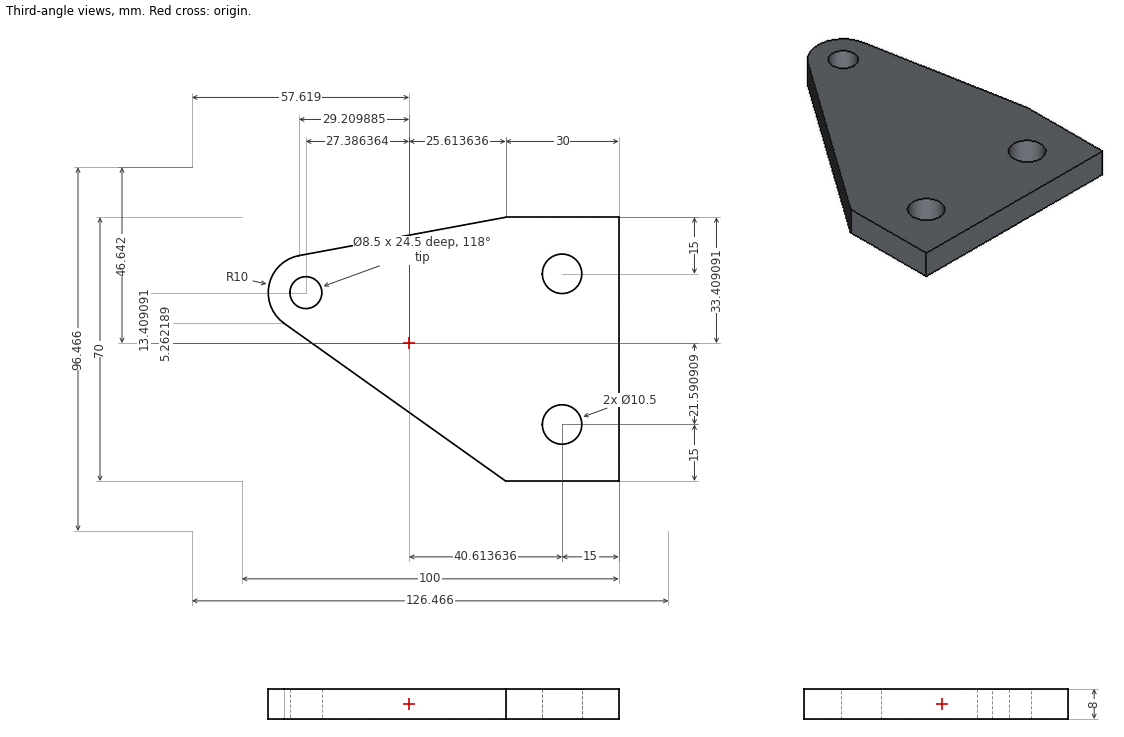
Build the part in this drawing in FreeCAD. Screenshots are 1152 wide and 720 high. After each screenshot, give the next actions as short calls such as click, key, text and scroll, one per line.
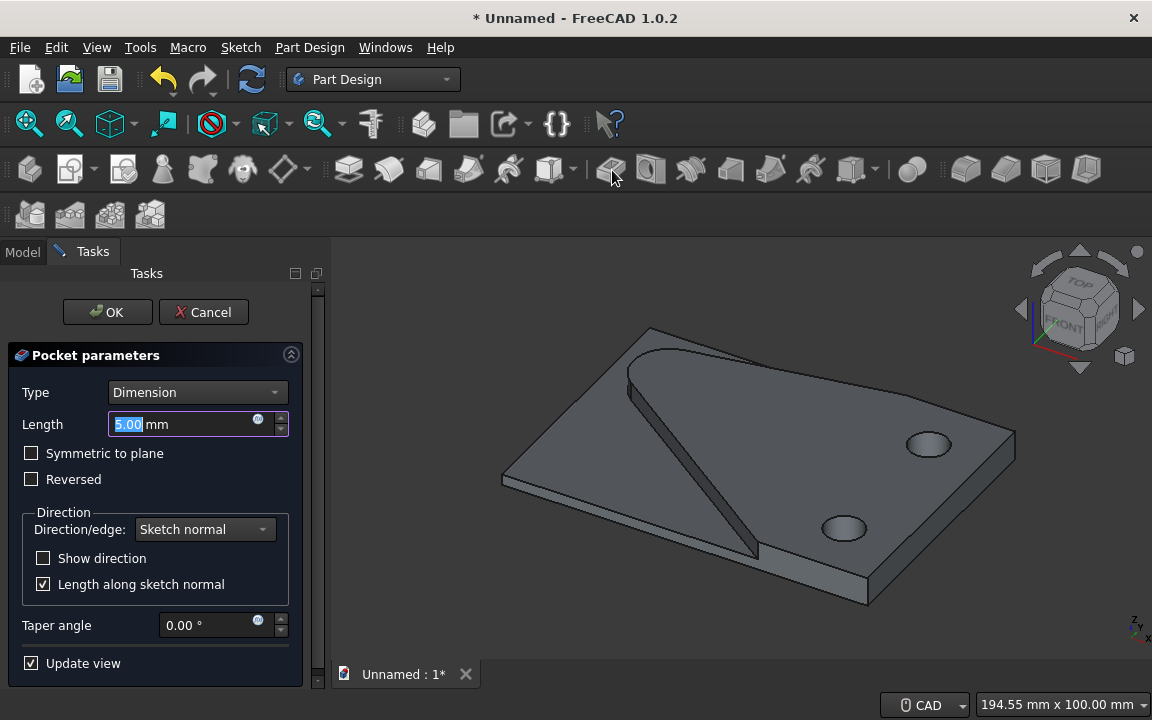
text(10)
key(Tab)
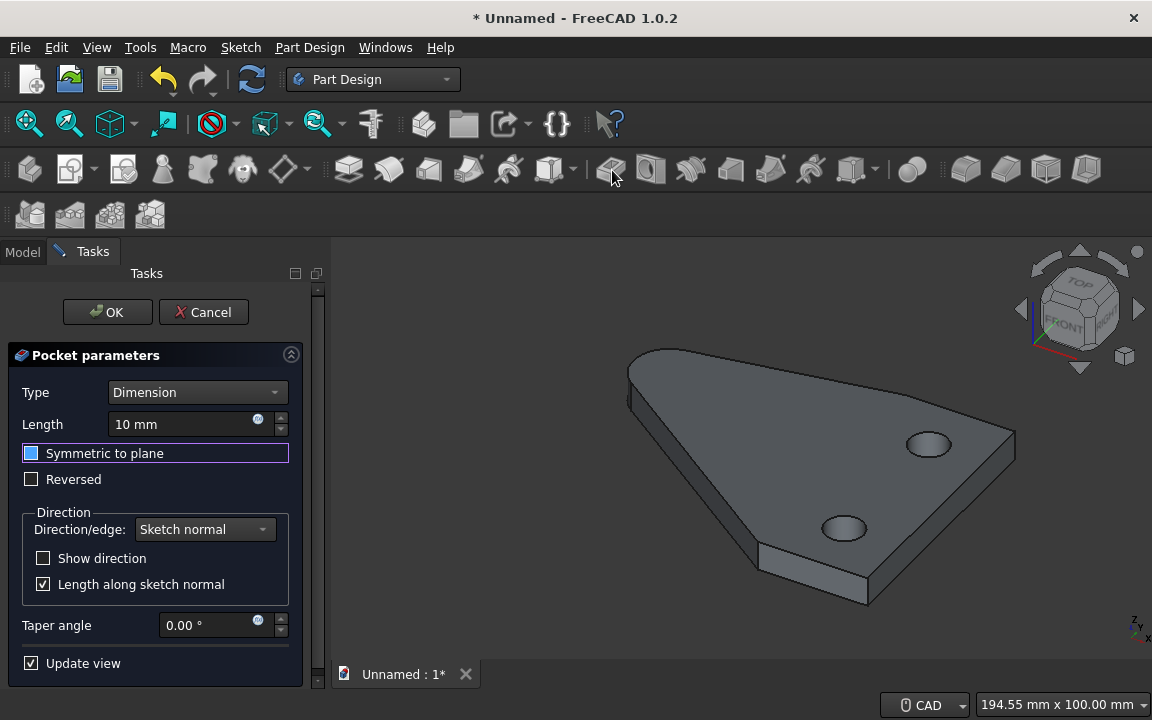
click(108, 312)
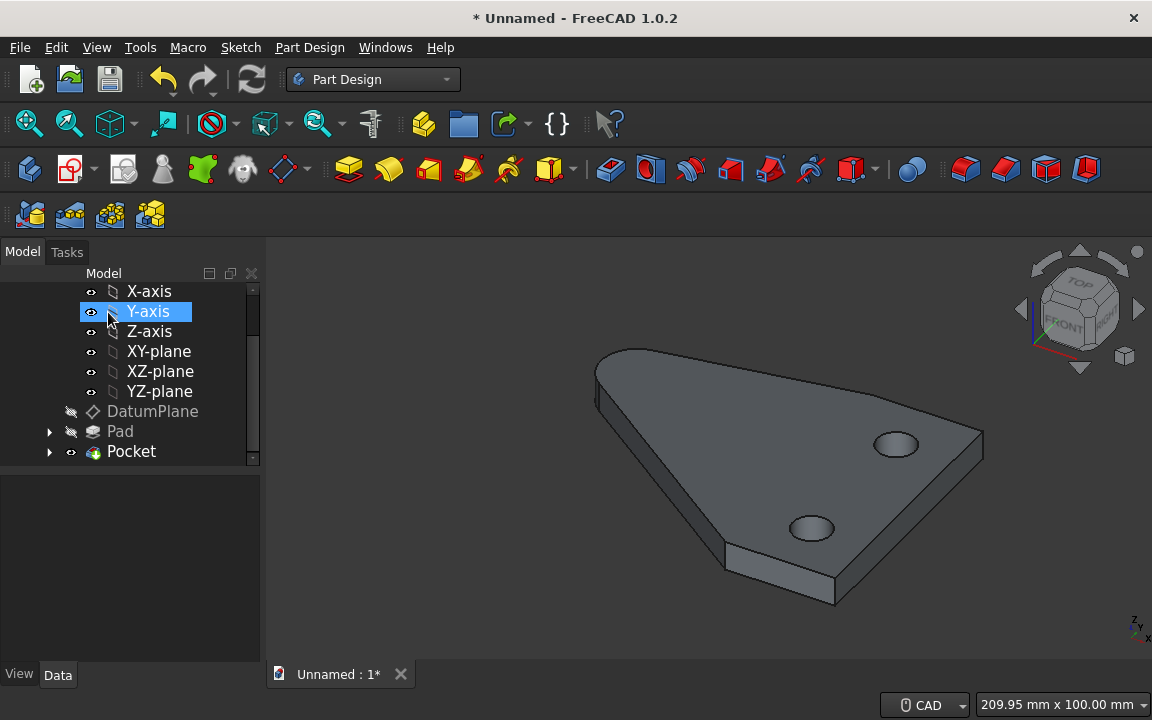
click(788, 464)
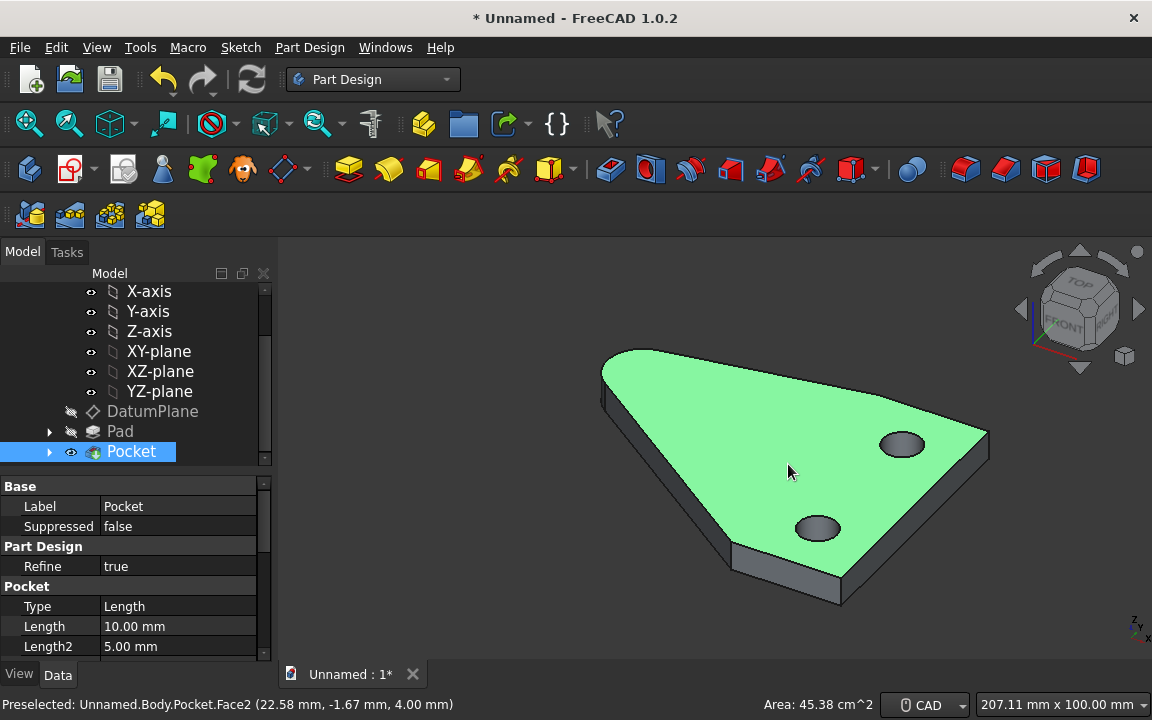
click(70, 170)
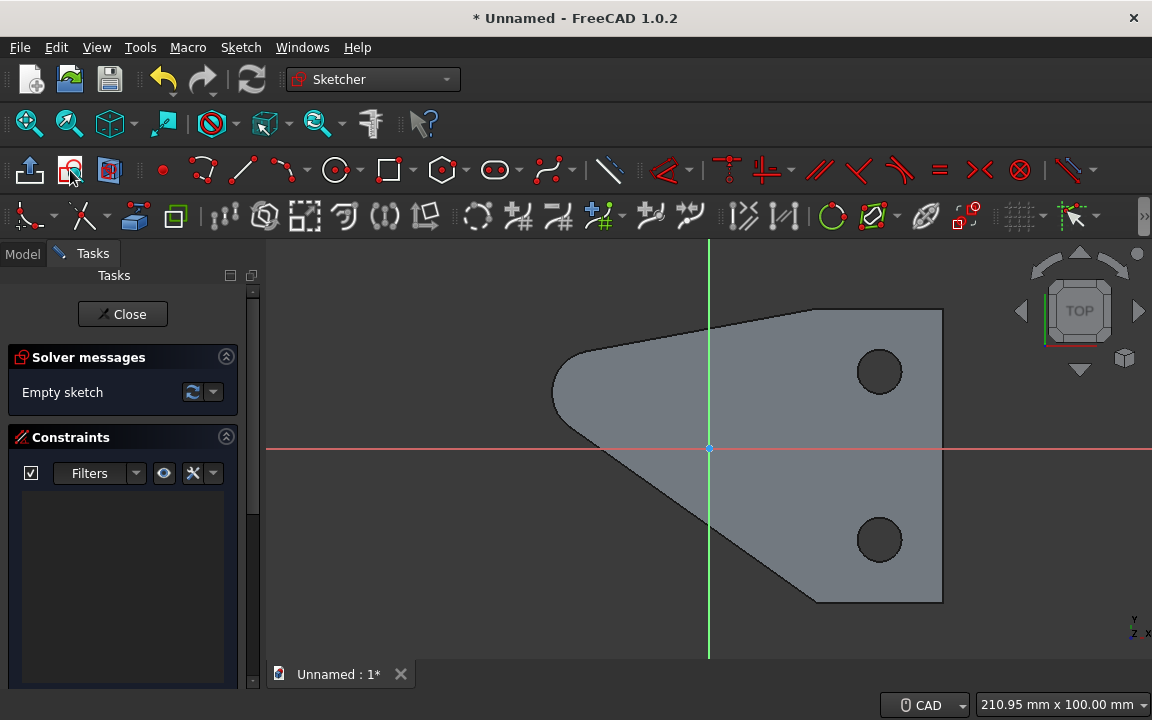
scroll(587, 384, up, 10)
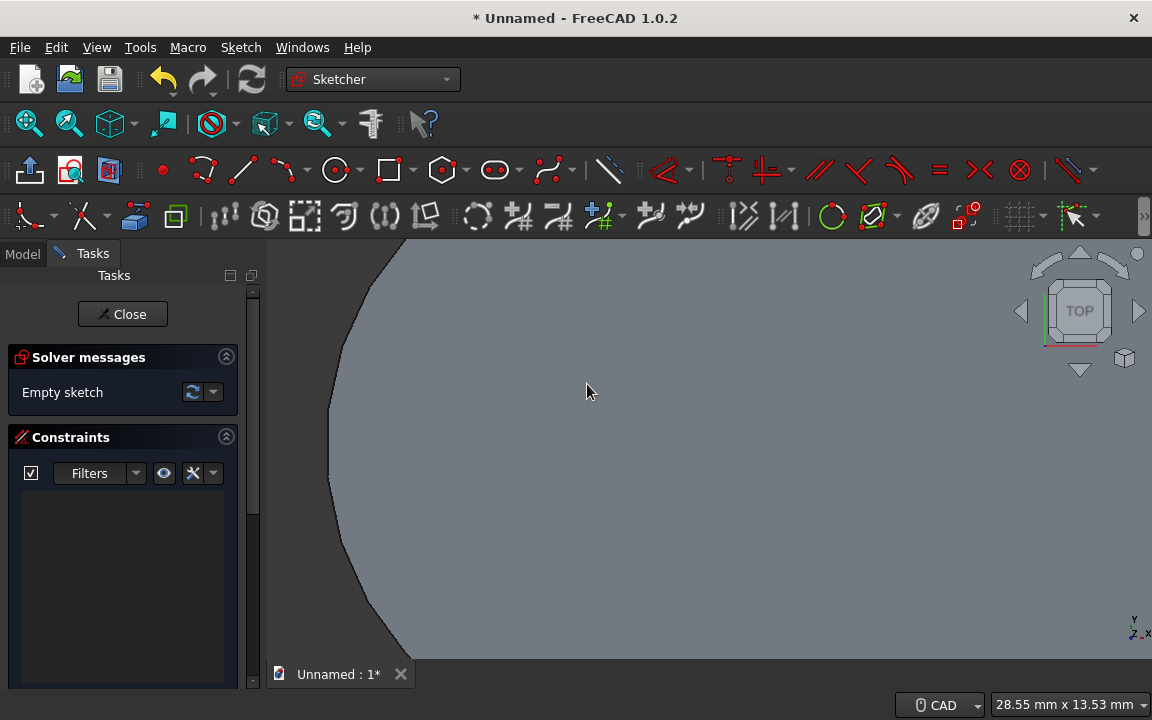
click(336, 170)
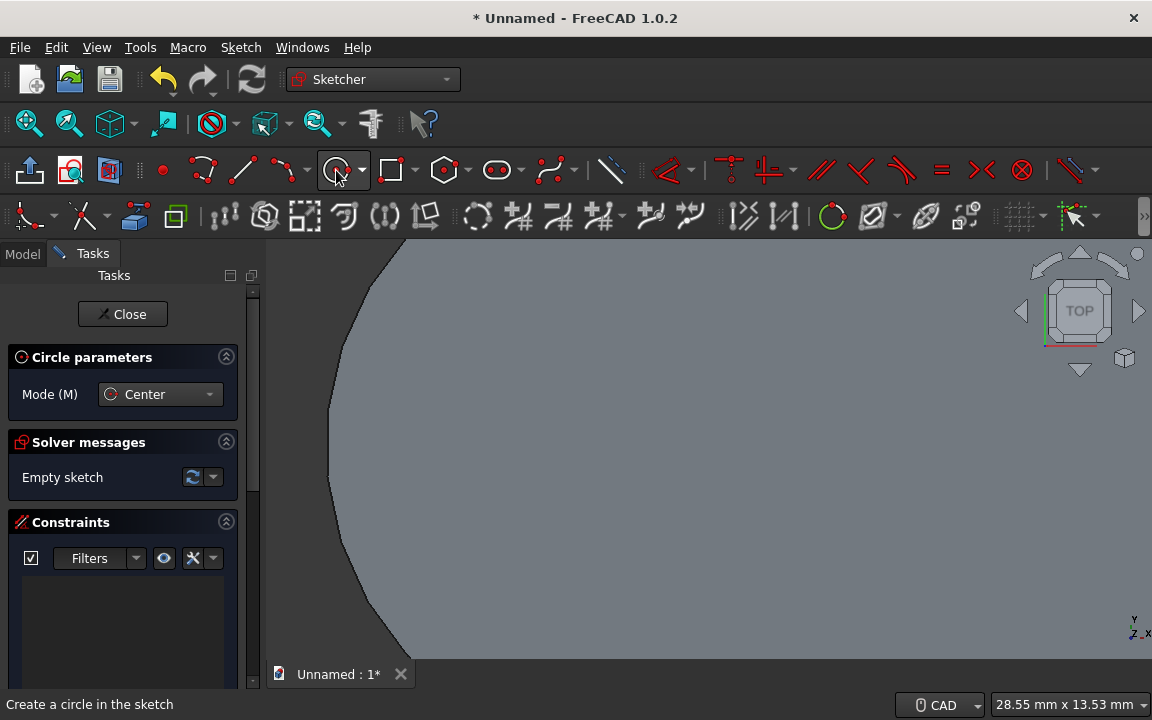
click(636, 446)
click(730, 353)
key(Escape)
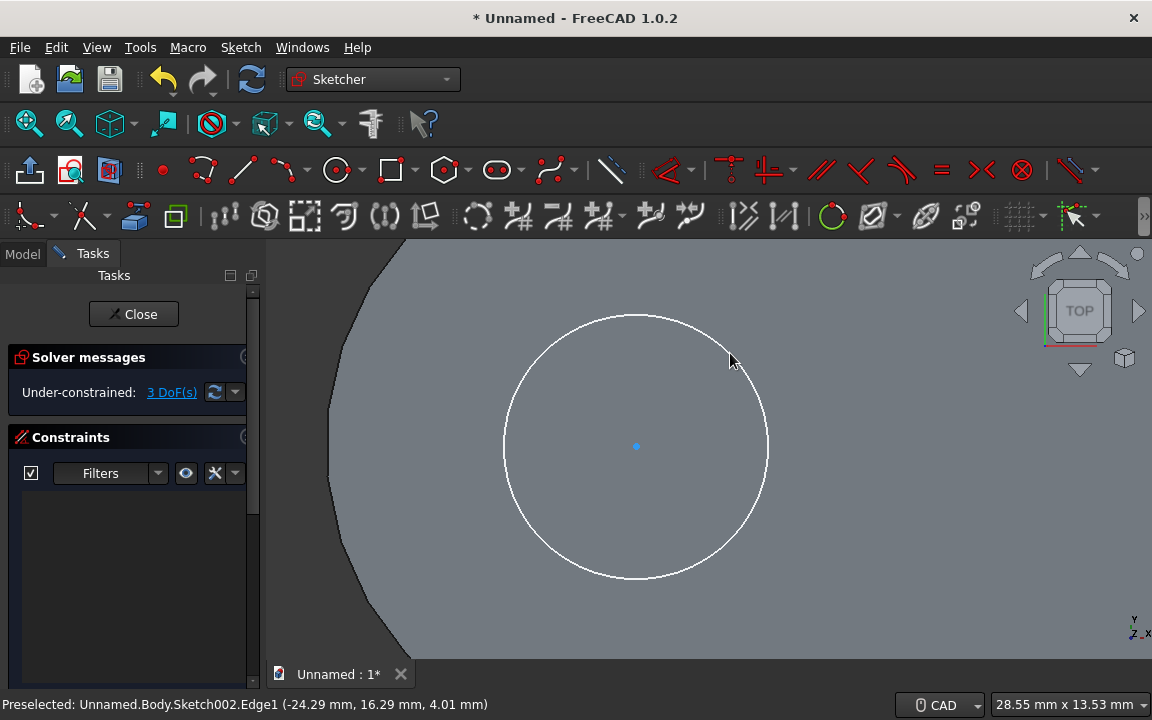
click(666, 170)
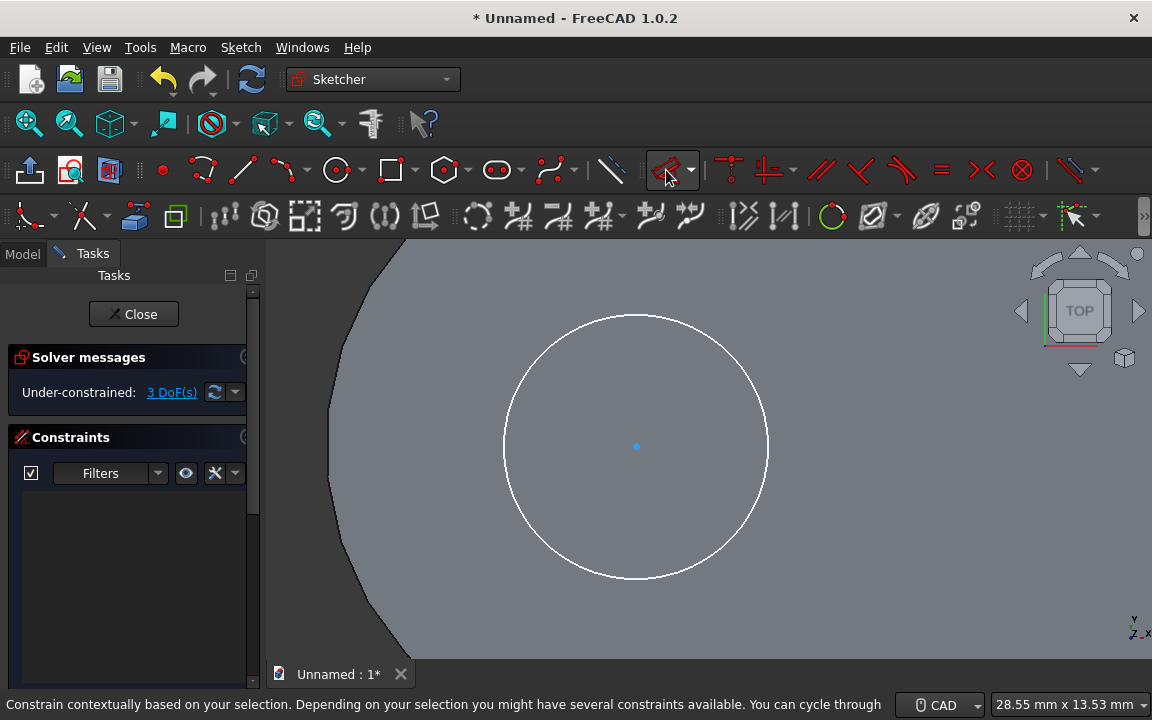
click(729, 353)
click(752, 330)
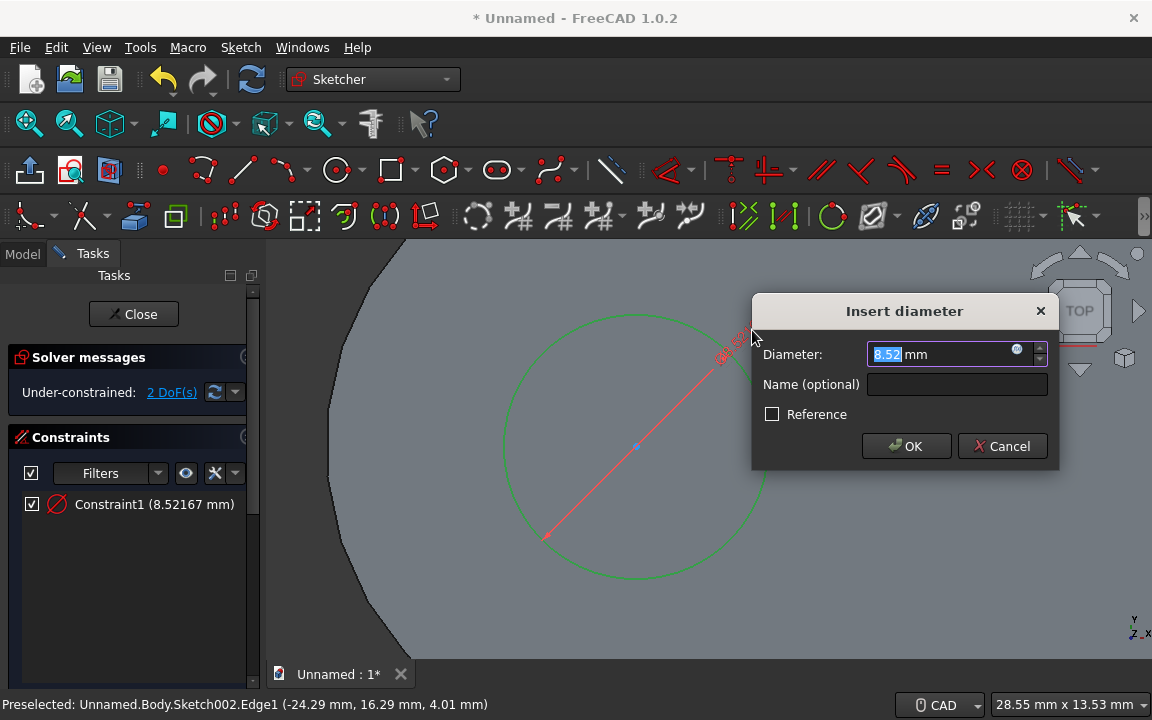
text(8.5)
key(Return)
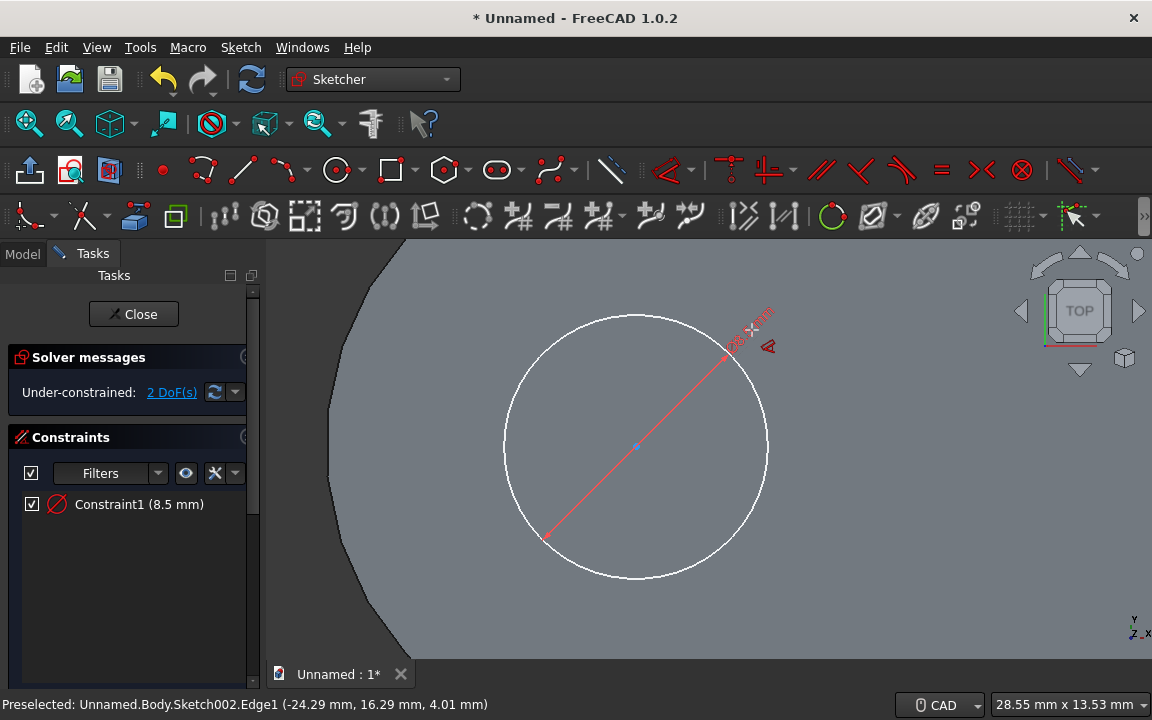
click(636, 447)
click(811, 413)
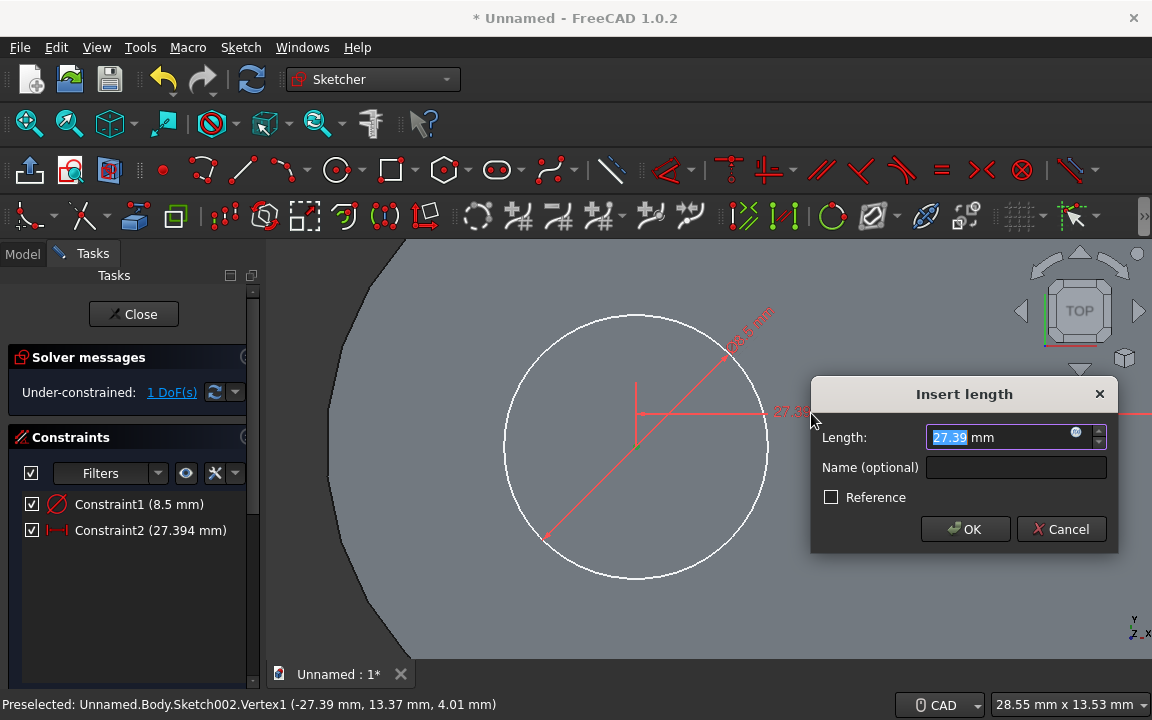
text(27.386364)
key(Return)